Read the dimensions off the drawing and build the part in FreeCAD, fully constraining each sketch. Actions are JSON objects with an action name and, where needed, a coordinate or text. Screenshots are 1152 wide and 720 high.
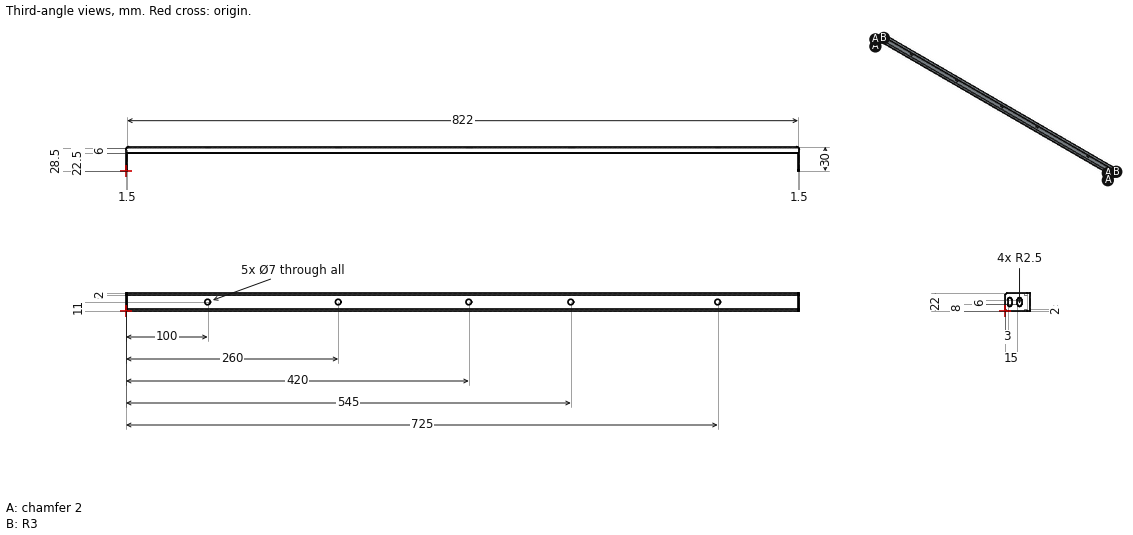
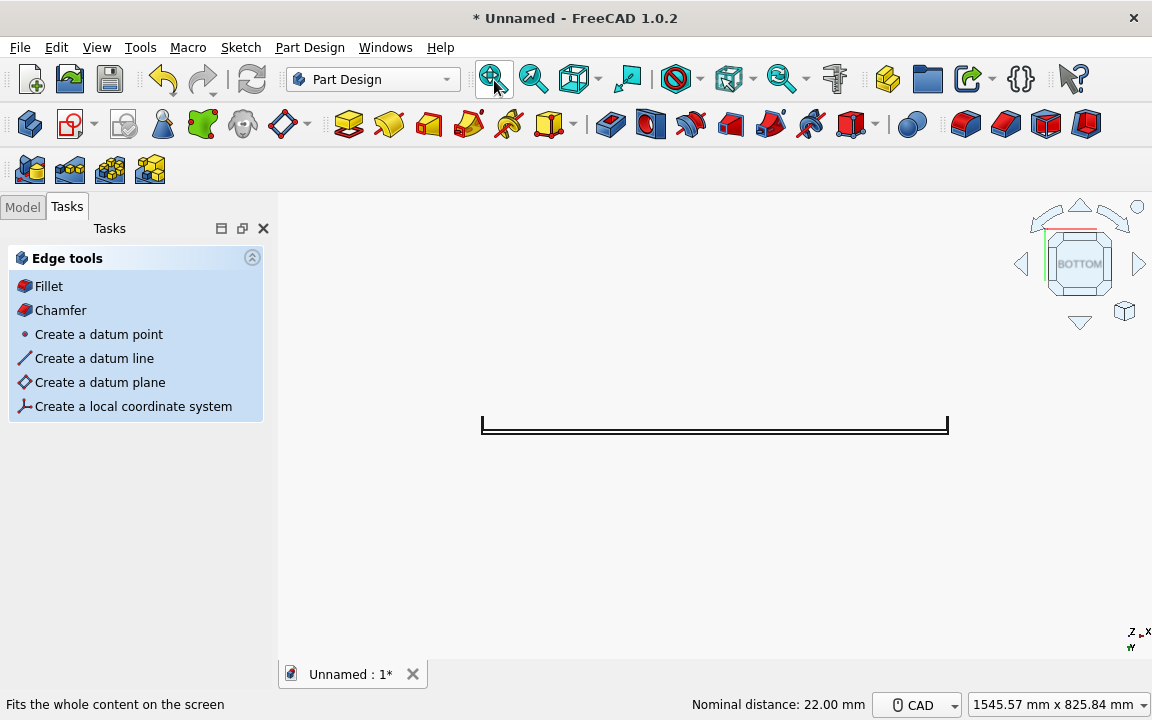
{"action": "scroll", "coordinate": [948, 416], "scroll_direction": "up", "scroll_amount": 15}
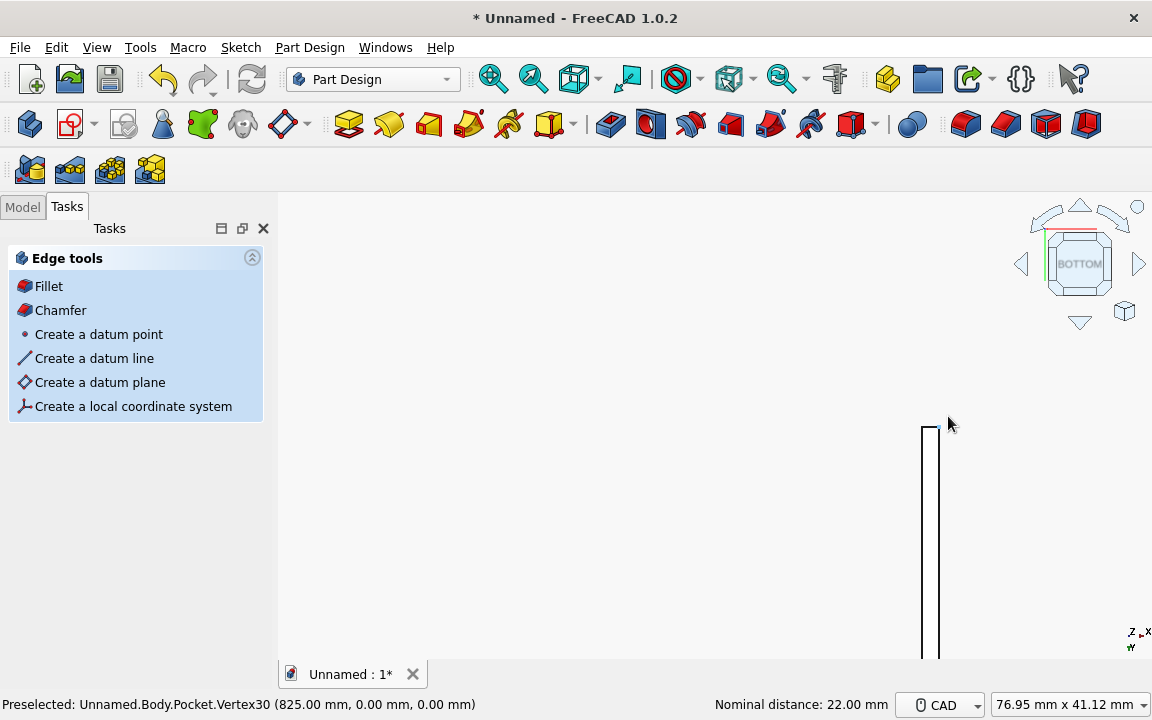
{"action": "left_click", "coordinate": [930, 426], "text": "ctrl"}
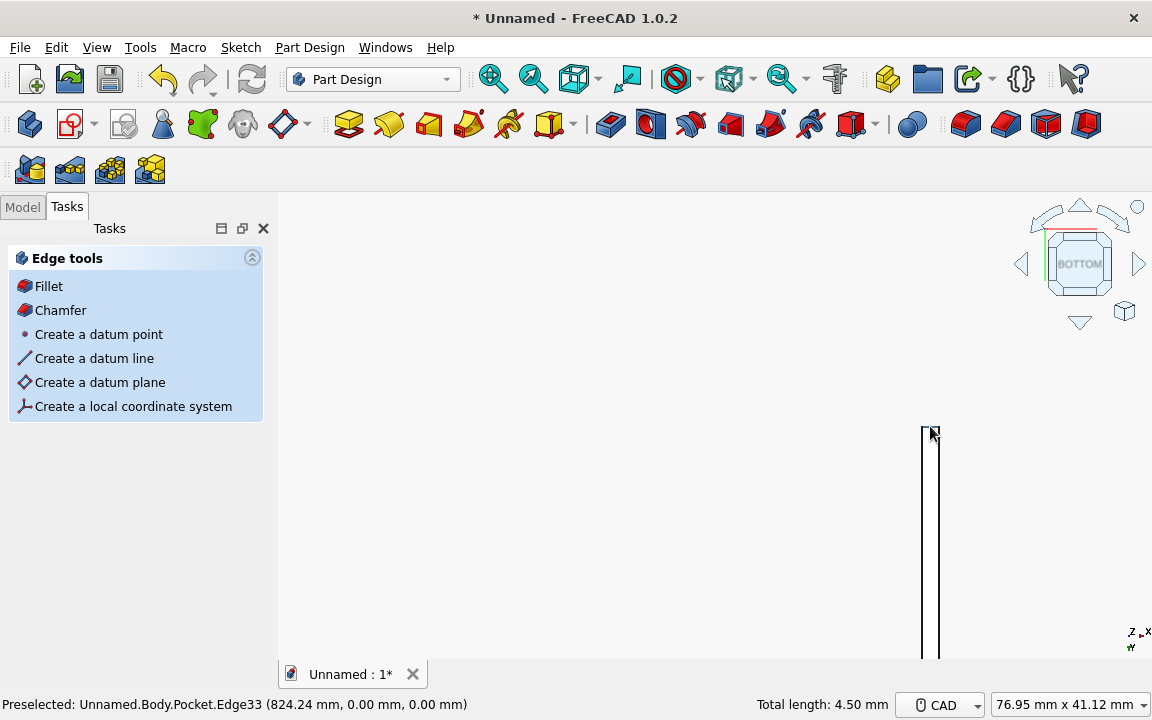
{"action": "scroll", "coordinate": [930, 426], "scroll_direction": "up", "scroll_amount": 5}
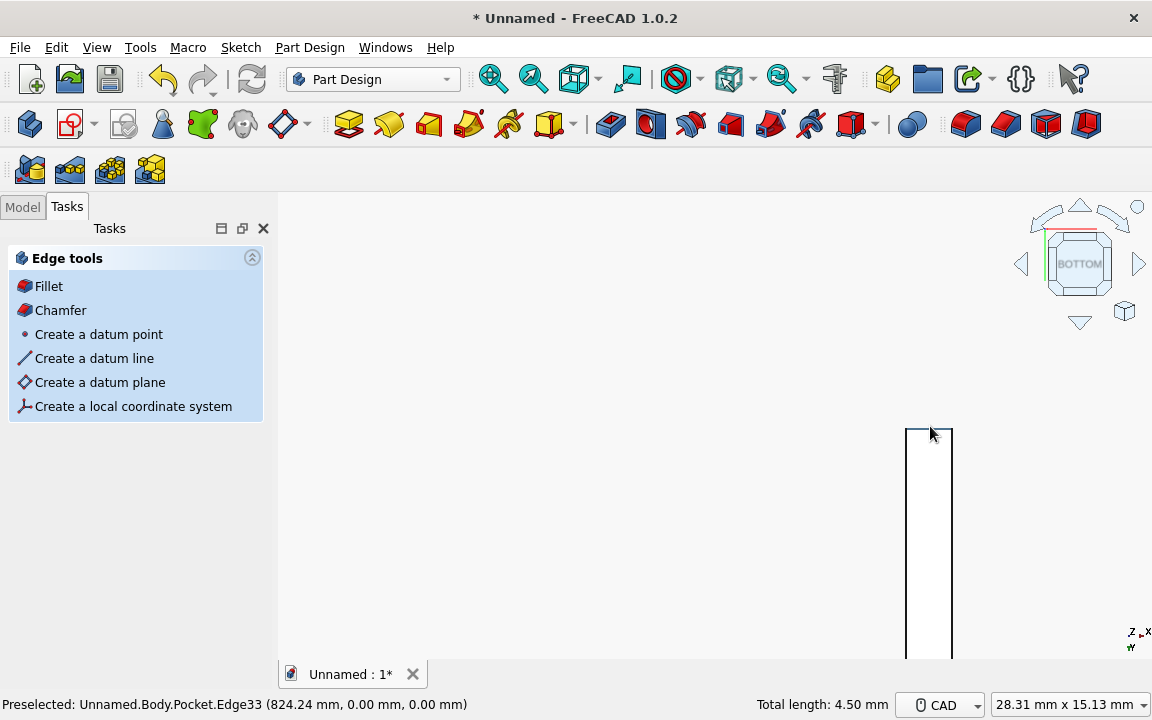
{"action": "left_click", "coordinate": [494, 80]}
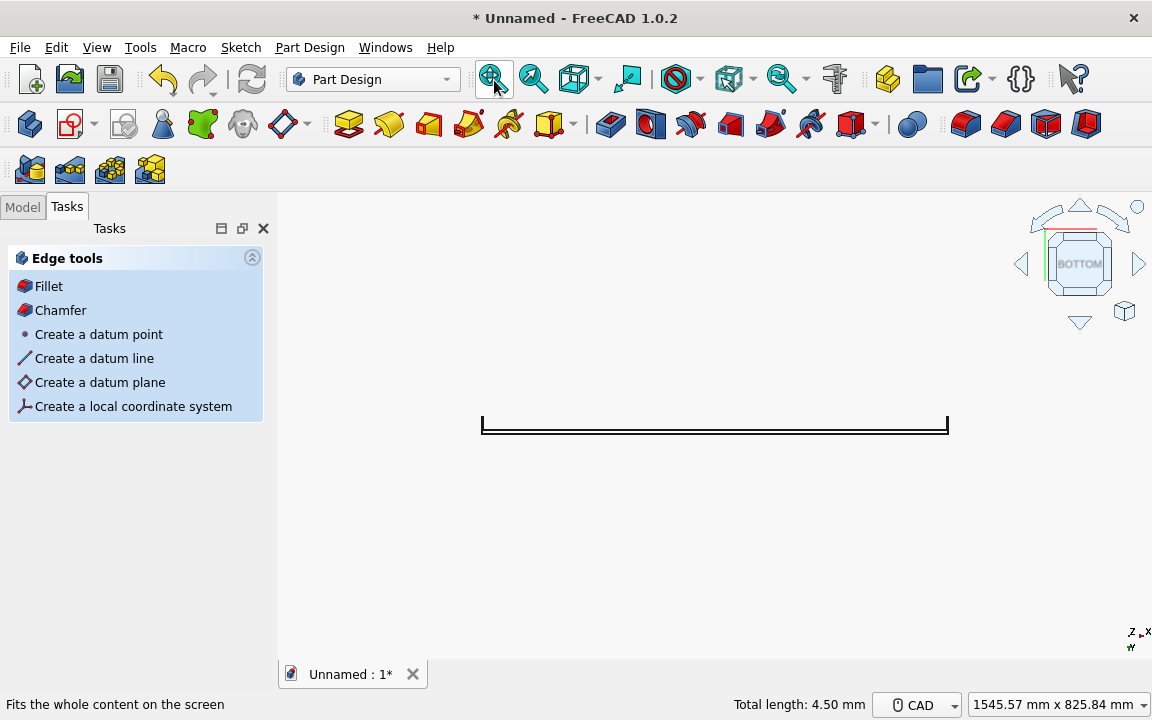
{"action": "key", "text": "4"}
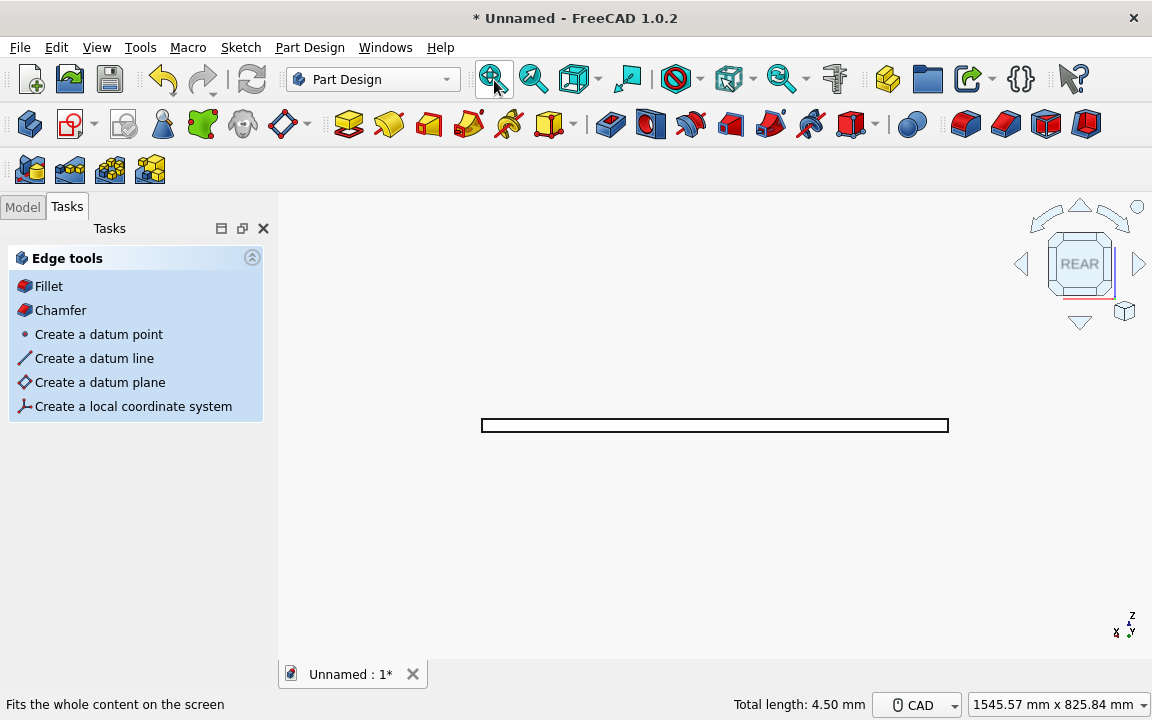
{"action": "scroll", "coordinate": [482, 418], "scroll_direction": "up", "scroll_amount": 15}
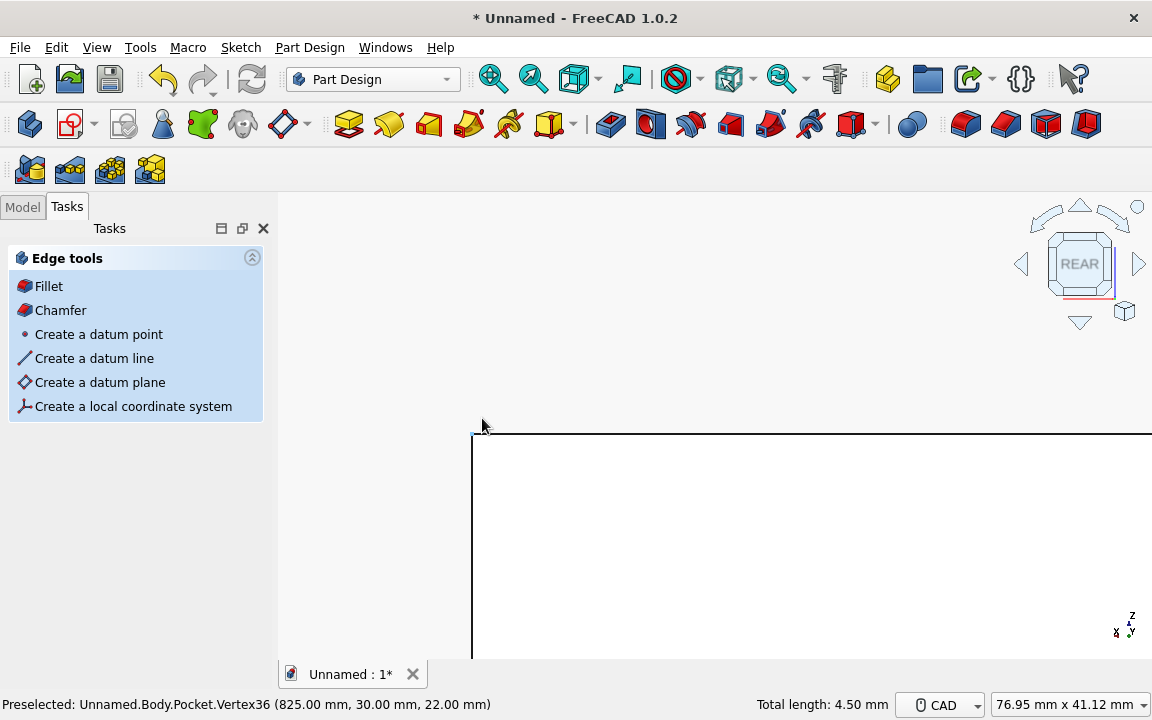
{"action": "scroll", "coordinate": [481, 433], "scroll_direction": "up", "scroll_amount": 5}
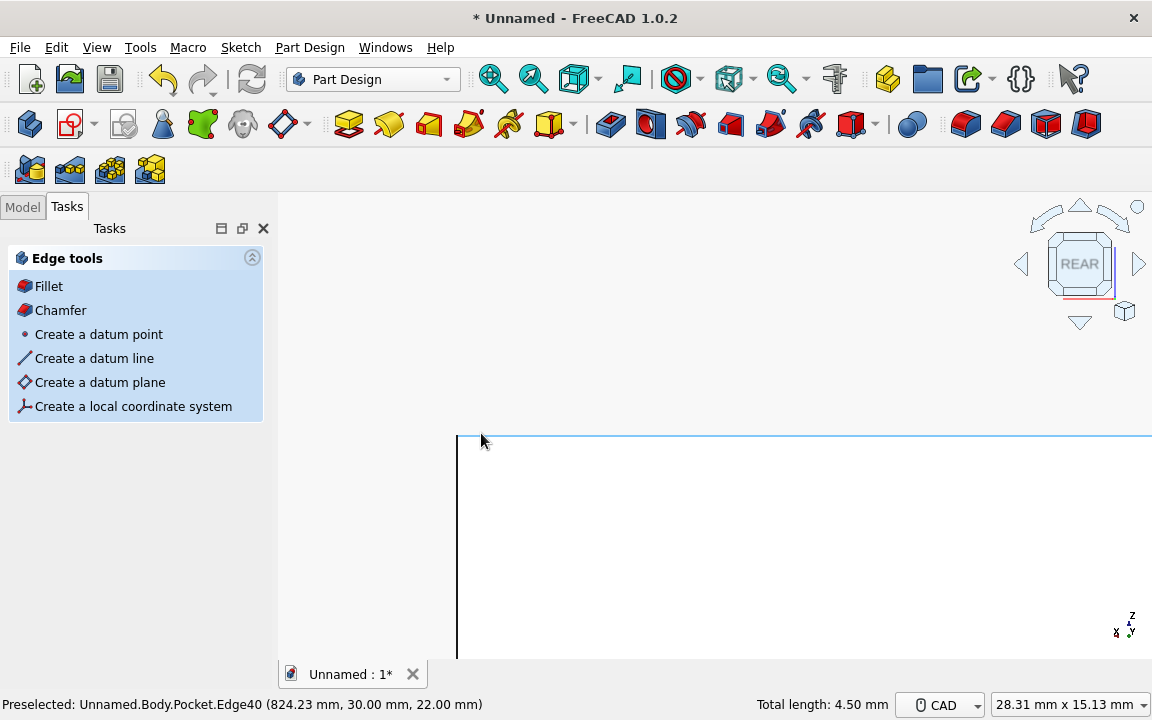
{"action": "left_click", "coordinate": [494, 80]}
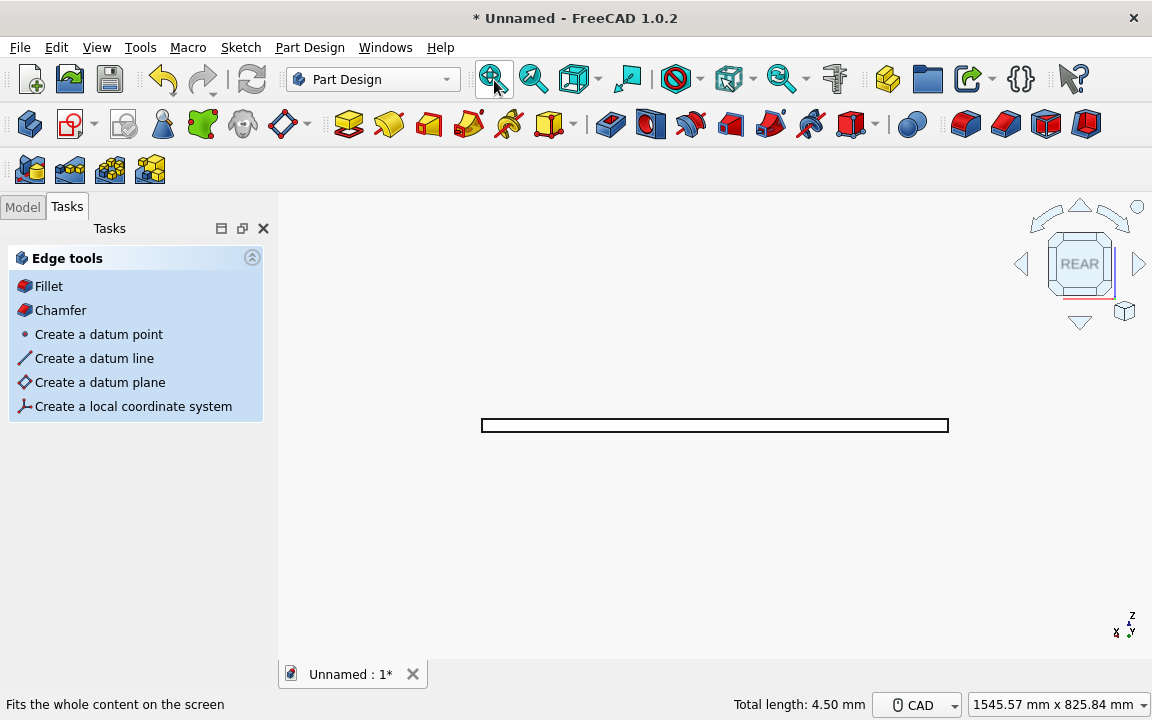
{"action": "key", "text": "6"}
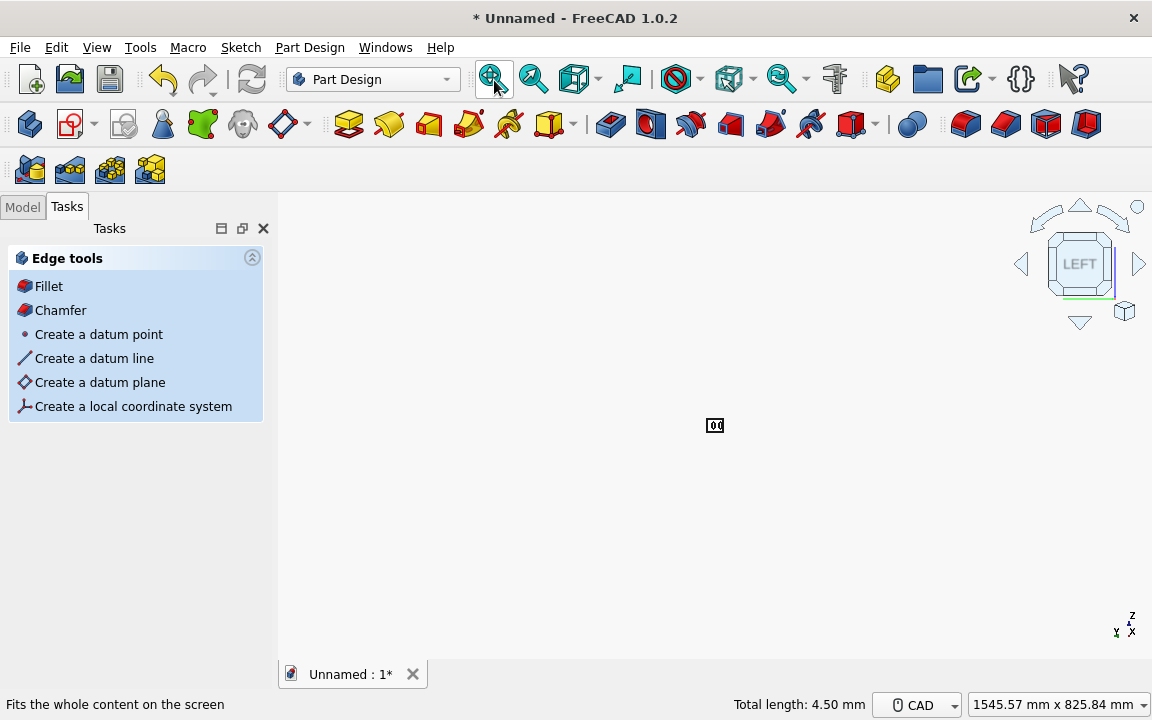
{"action": "left_click", "coordinate": [494, 80]}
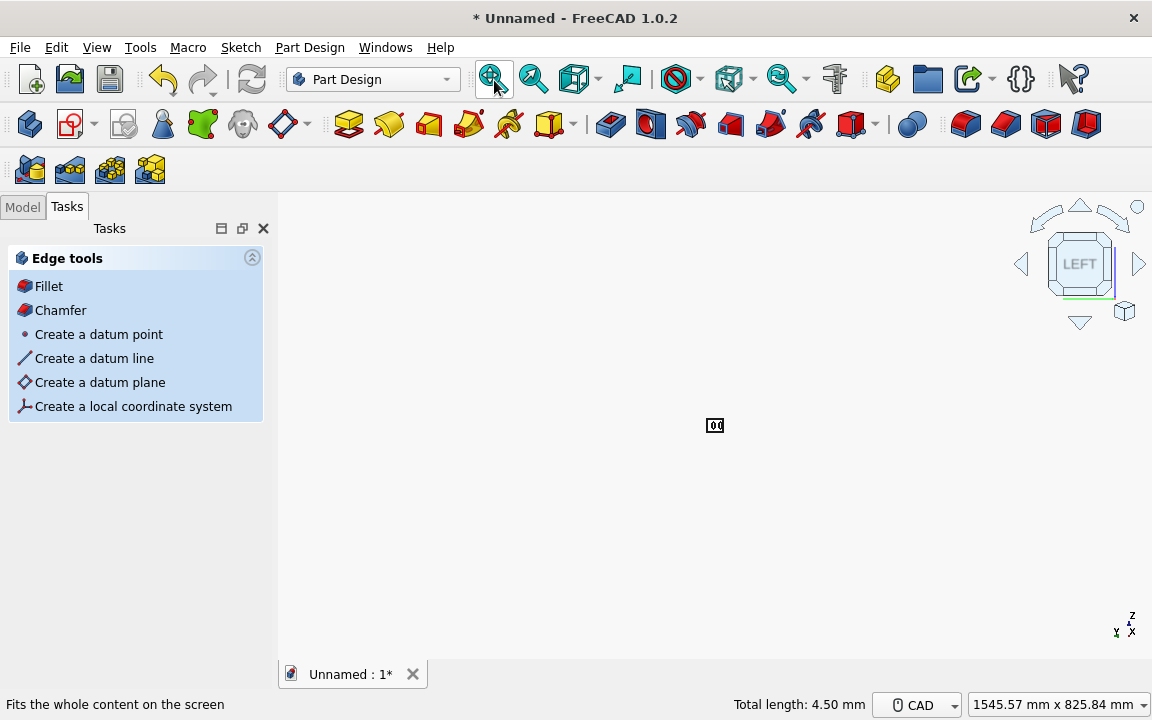
{"action": "scroll", "coordinate": [723, 418], "scroll_direction": "up", "scroll_amount": 15}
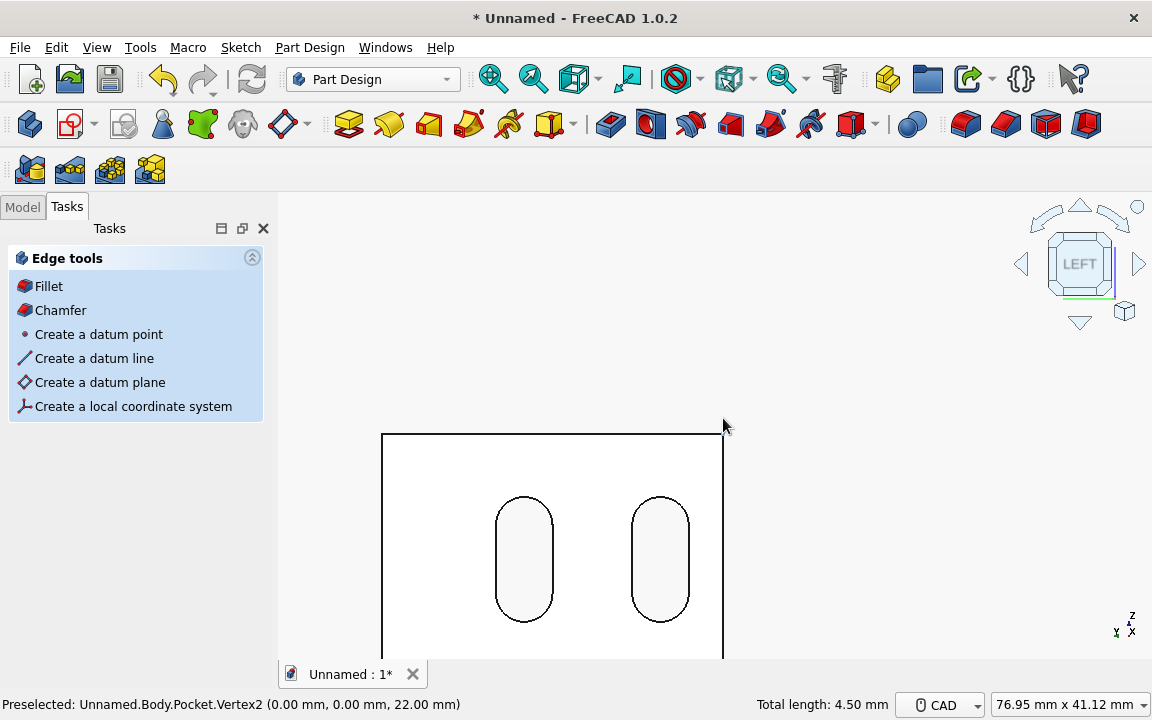
{"action": "scroll", "coordinate": [723, 433], "scroll_direction": "up", "scroll_amount": 5}